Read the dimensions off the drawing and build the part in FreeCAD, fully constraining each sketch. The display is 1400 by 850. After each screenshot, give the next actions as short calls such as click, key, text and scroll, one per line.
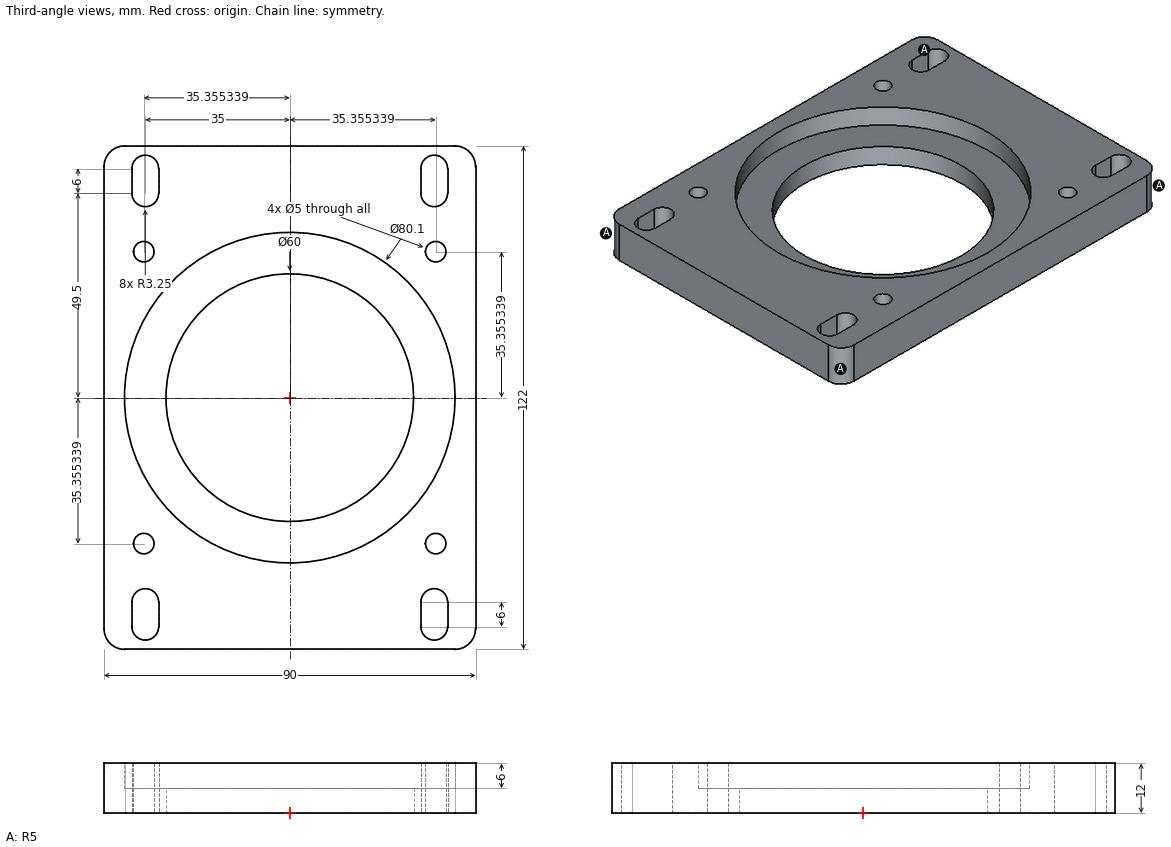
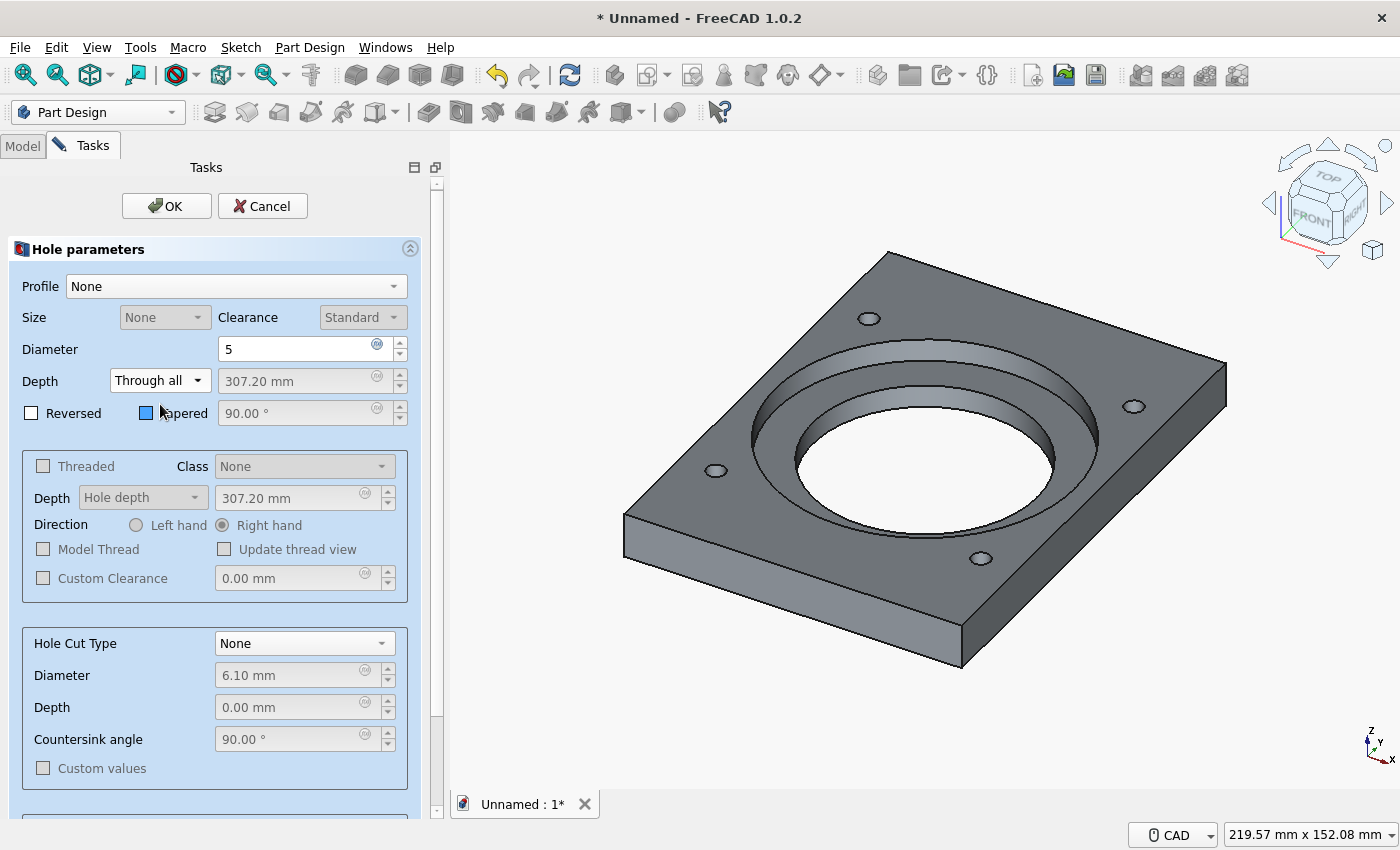
click(167, 206)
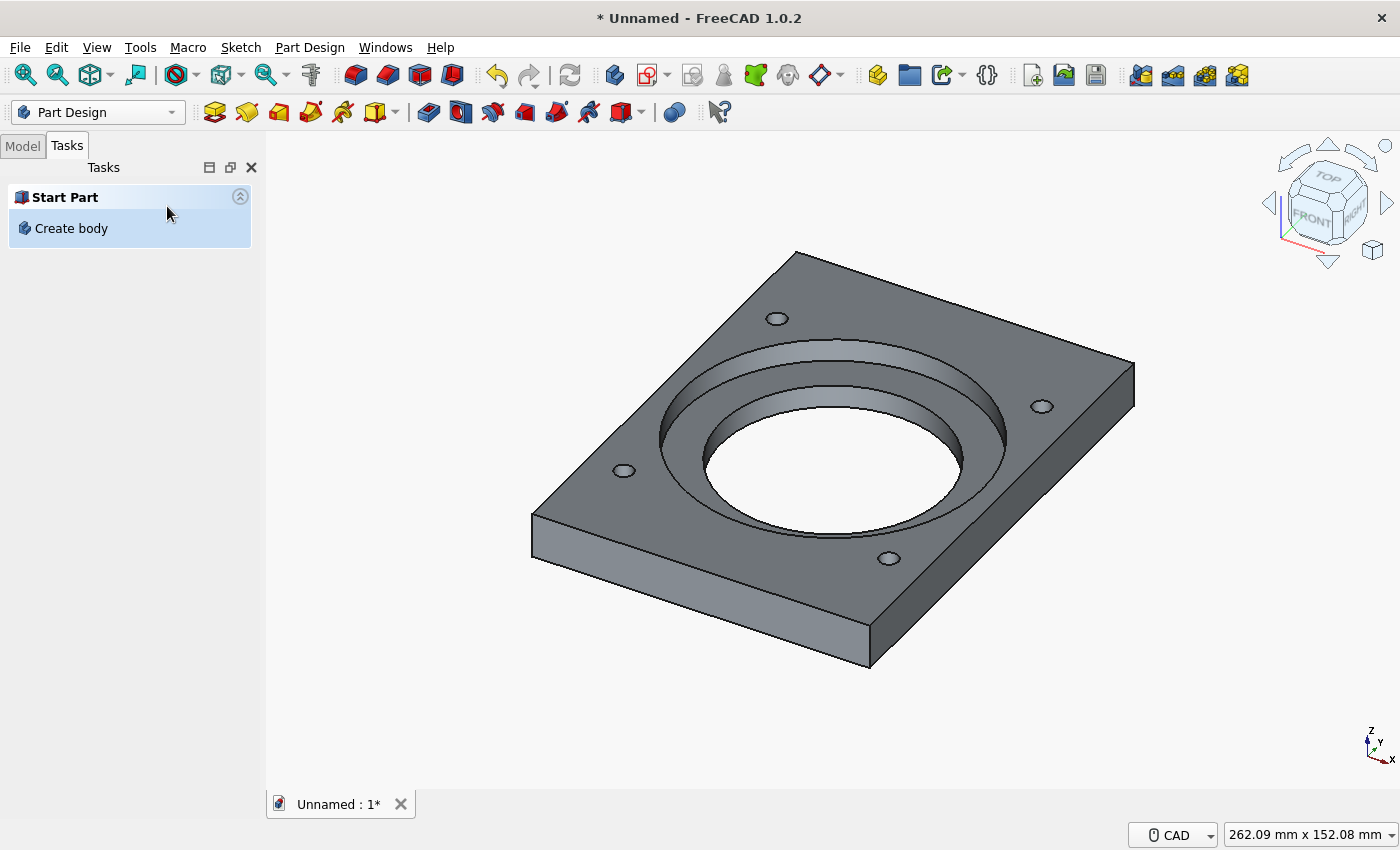
click(816, 582)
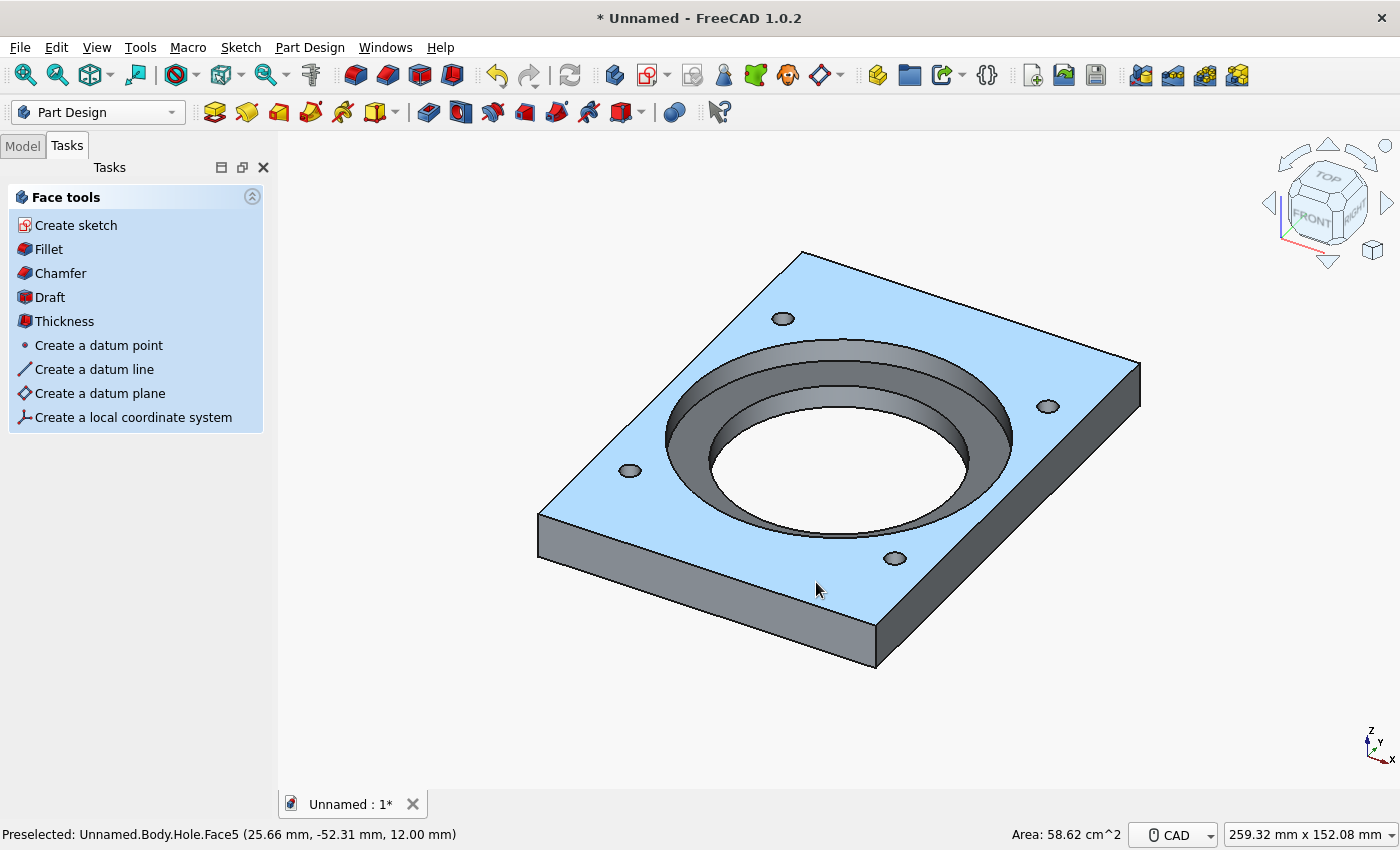
click(648, 76)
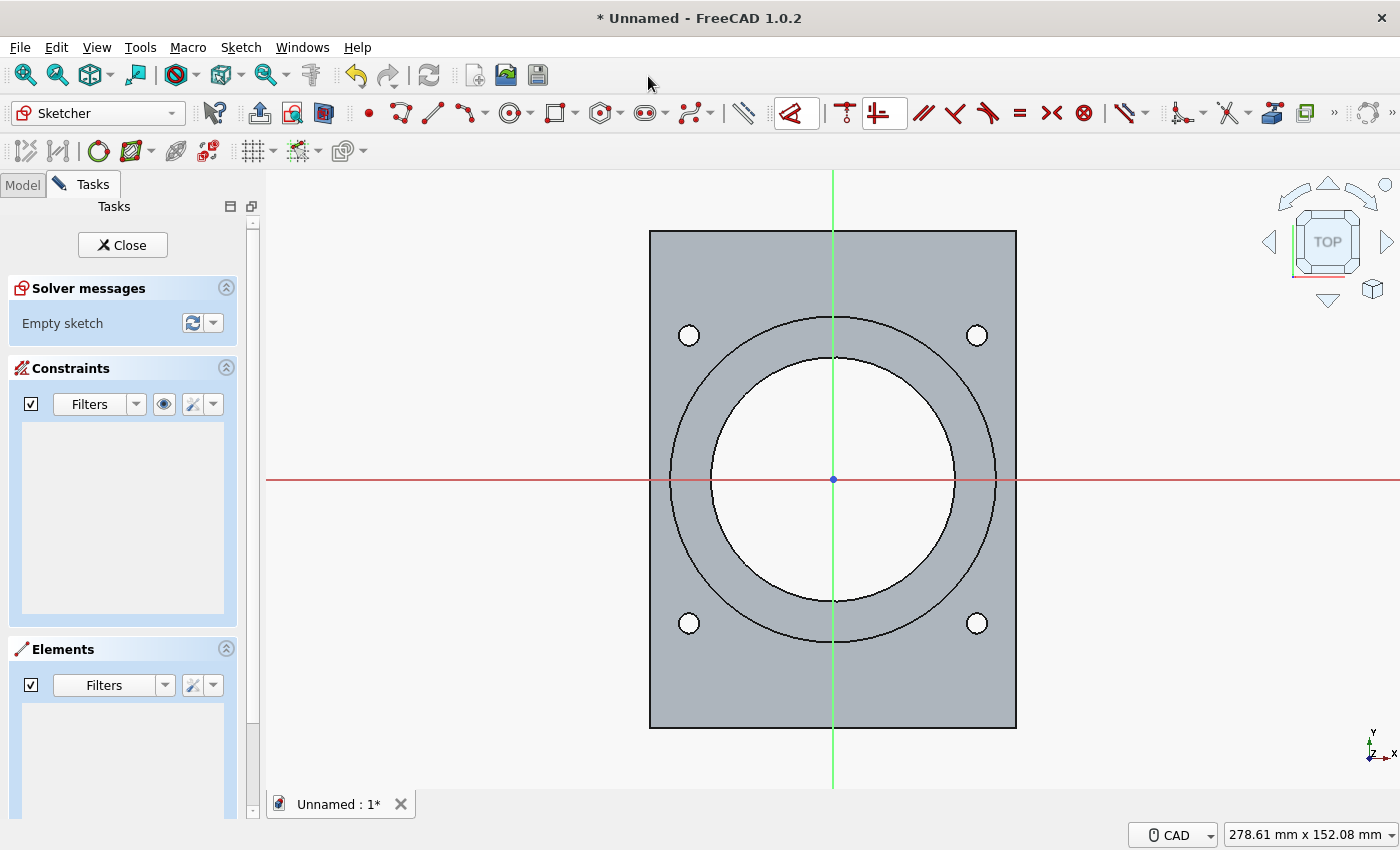
click(646, 114)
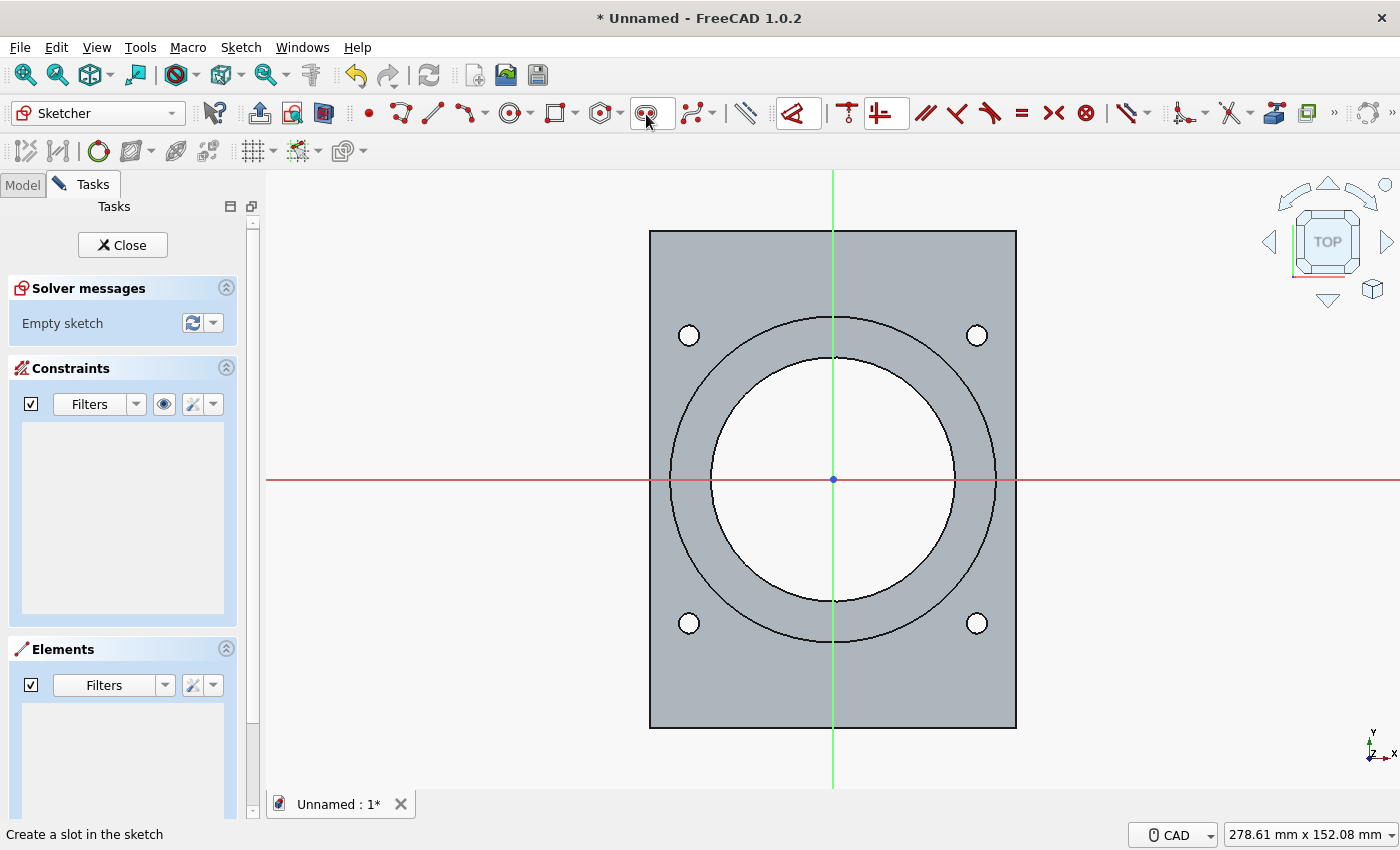
scroll(691, 278, up, 3)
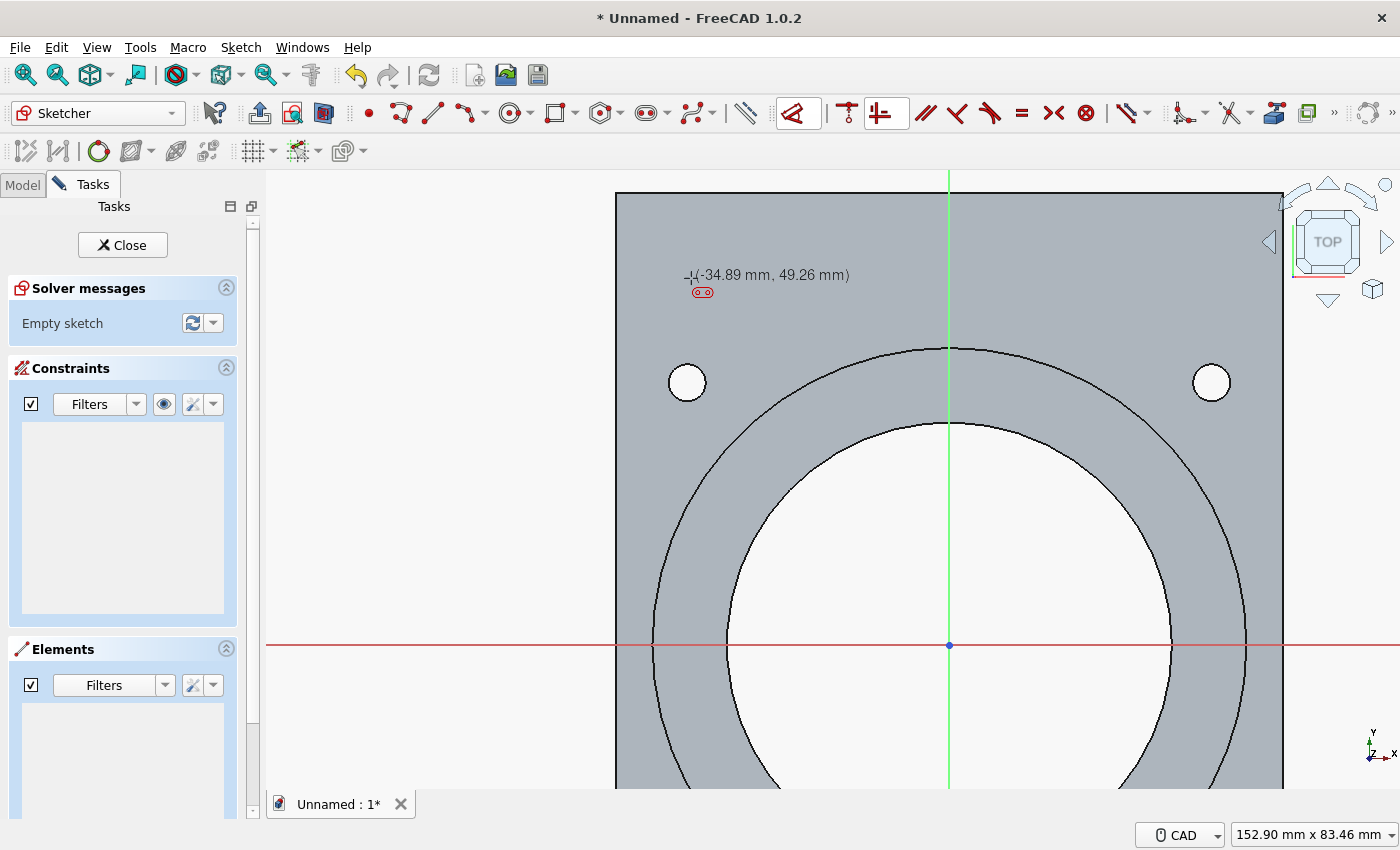
click(690, 278)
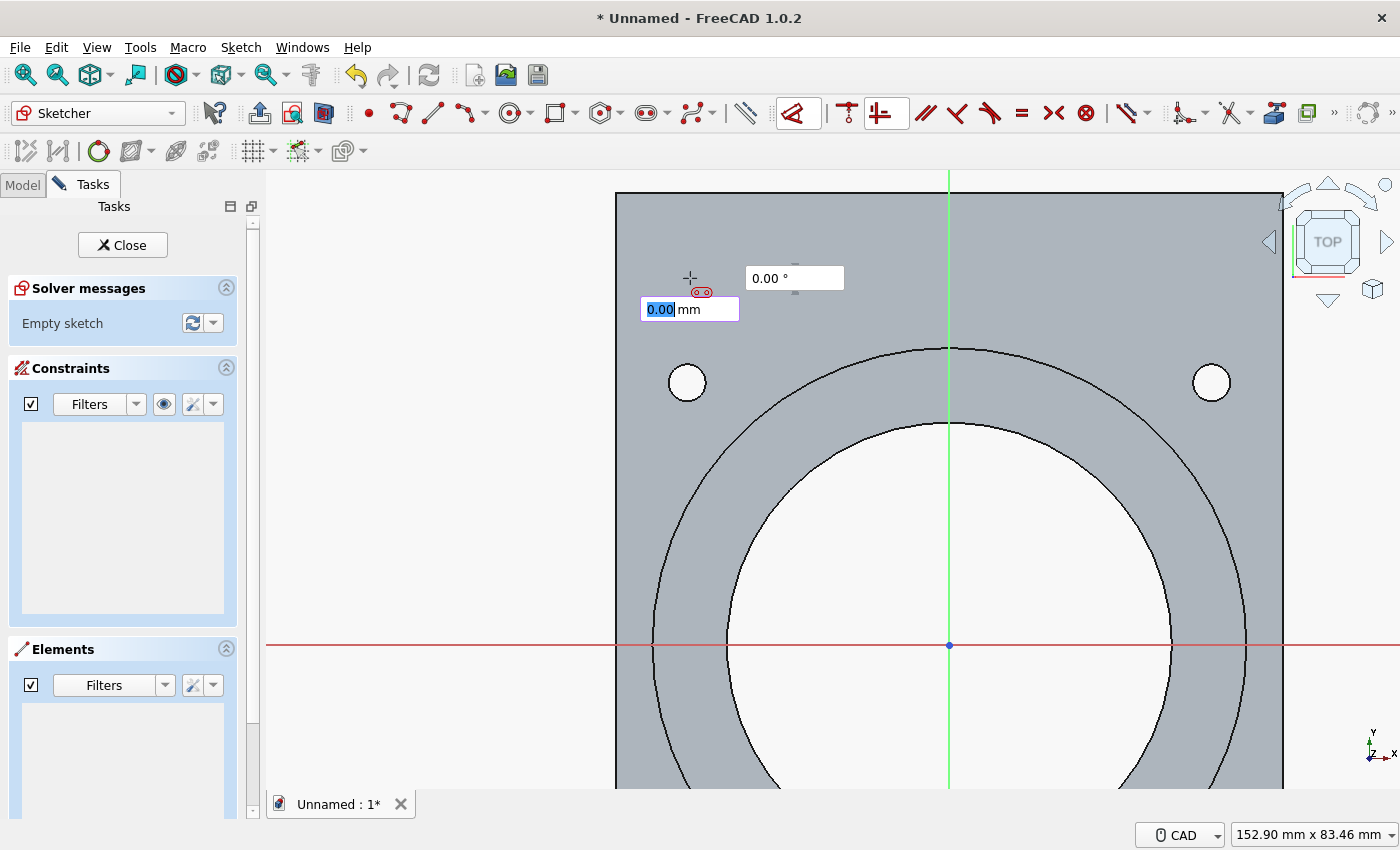
click(690, 233)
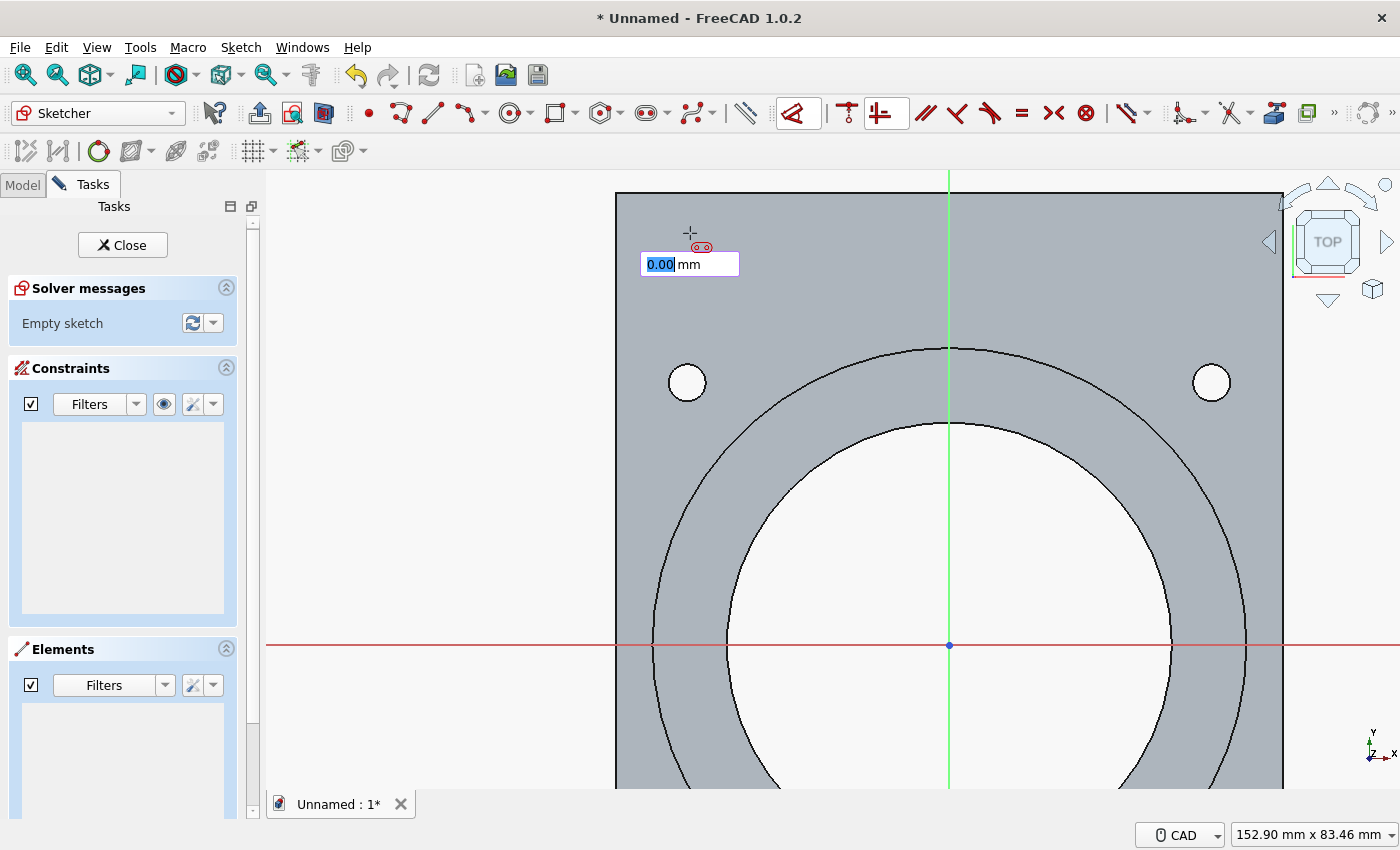
click(666, 256)